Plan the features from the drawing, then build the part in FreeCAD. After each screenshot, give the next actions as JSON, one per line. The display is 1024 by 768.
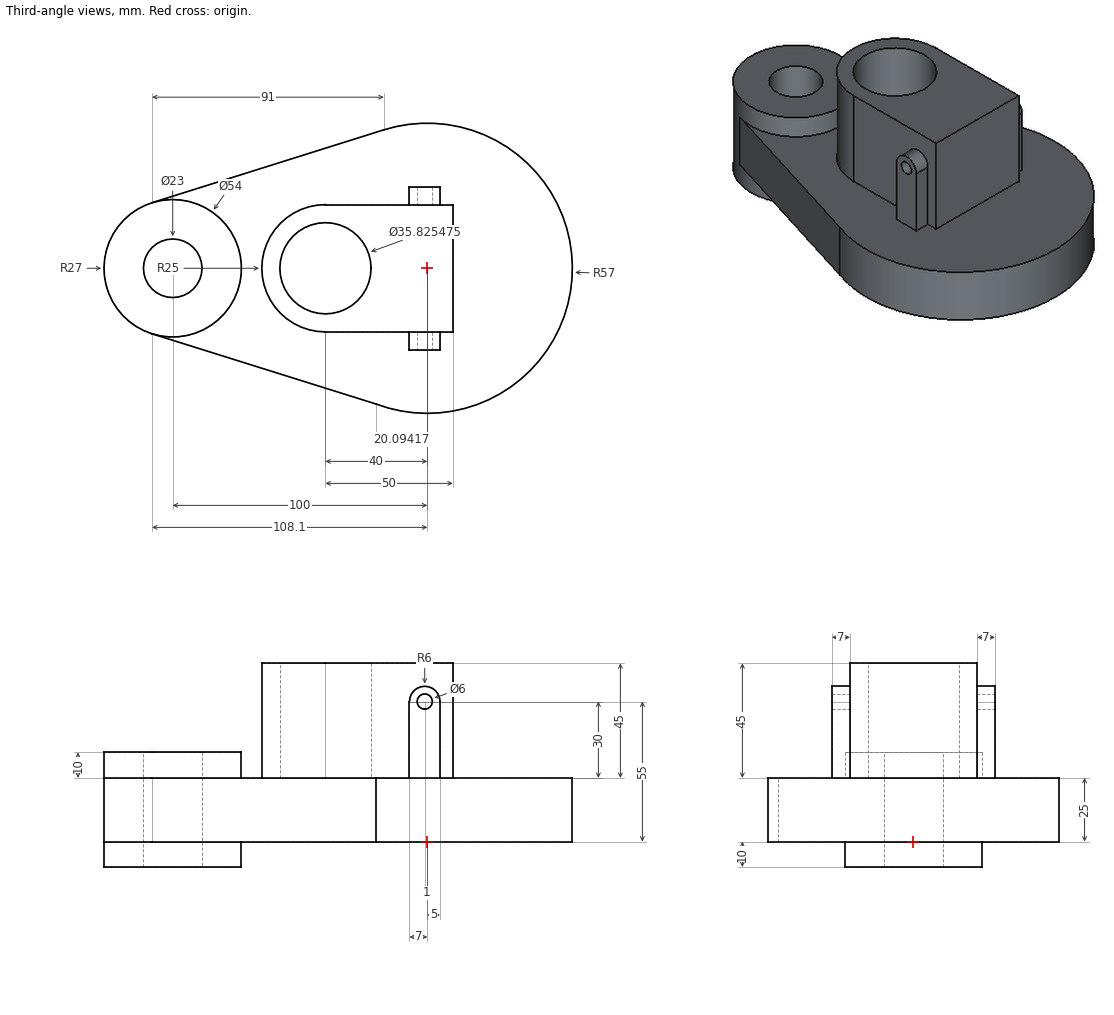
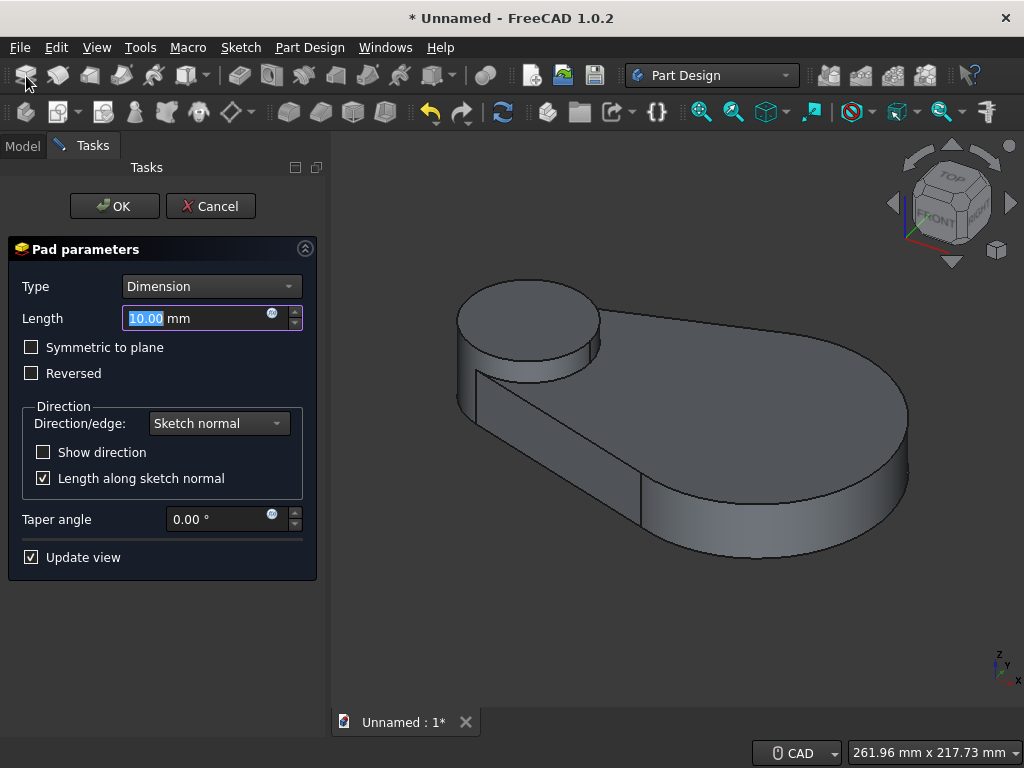
{"action": "type", "text": "10"}
{"action": "key", "text": "Tab"}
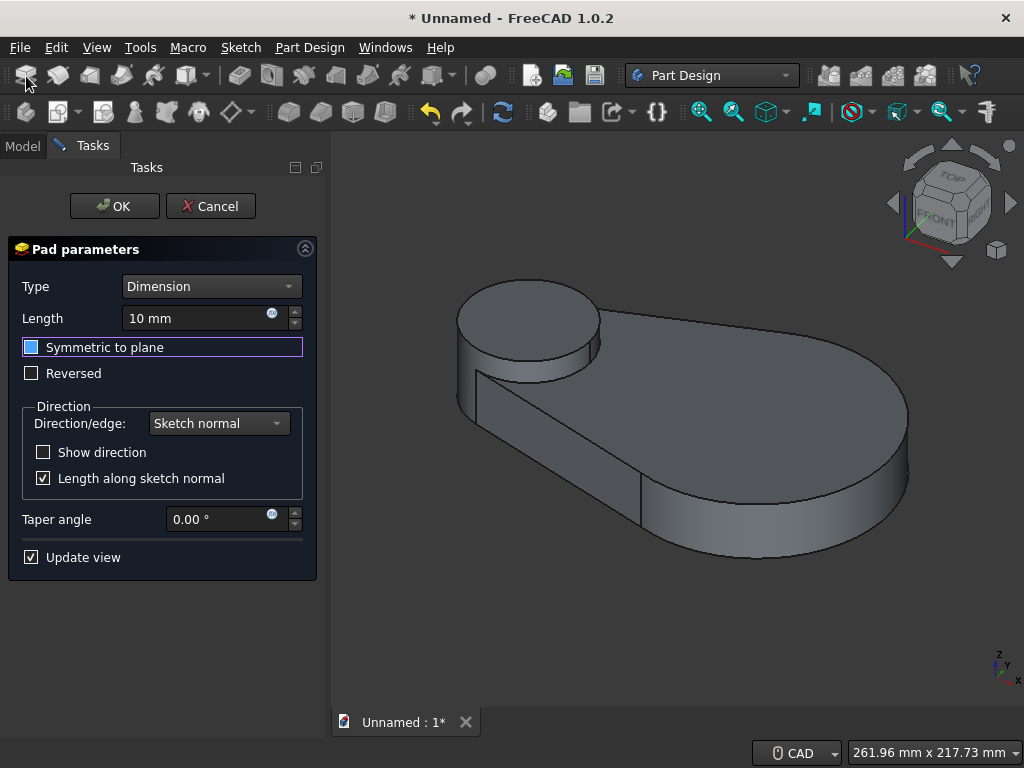
{"action": "left_click", "coordinate": [115, 206]}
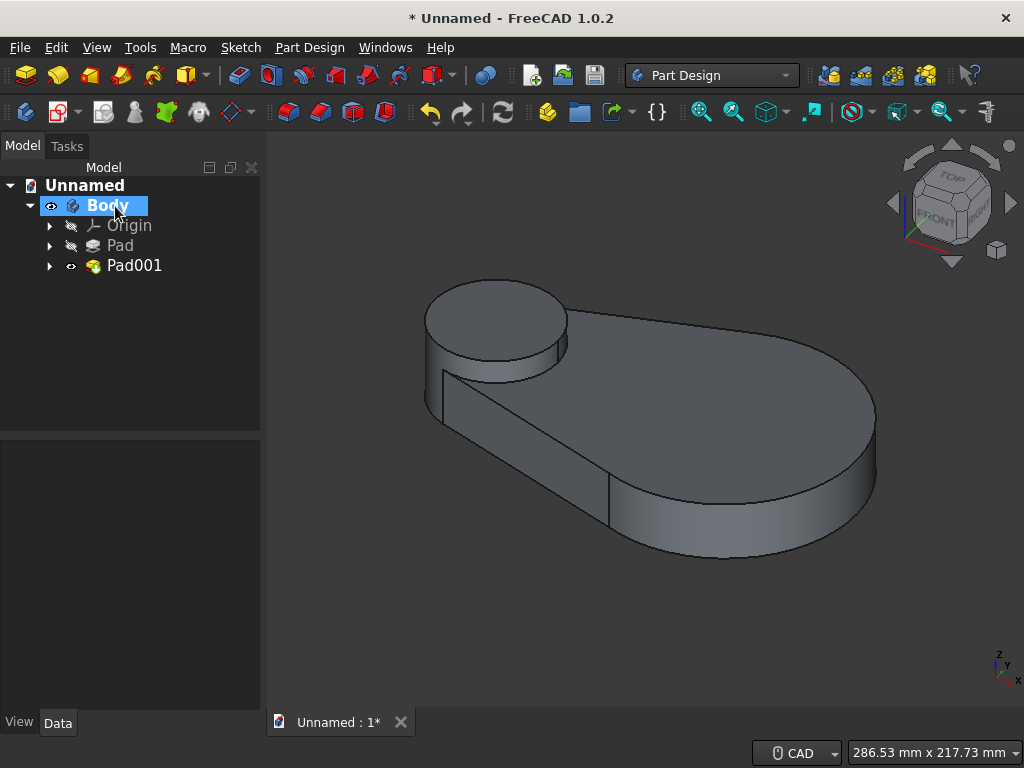
{"action": "left_click", "coordinate": [50, 226]}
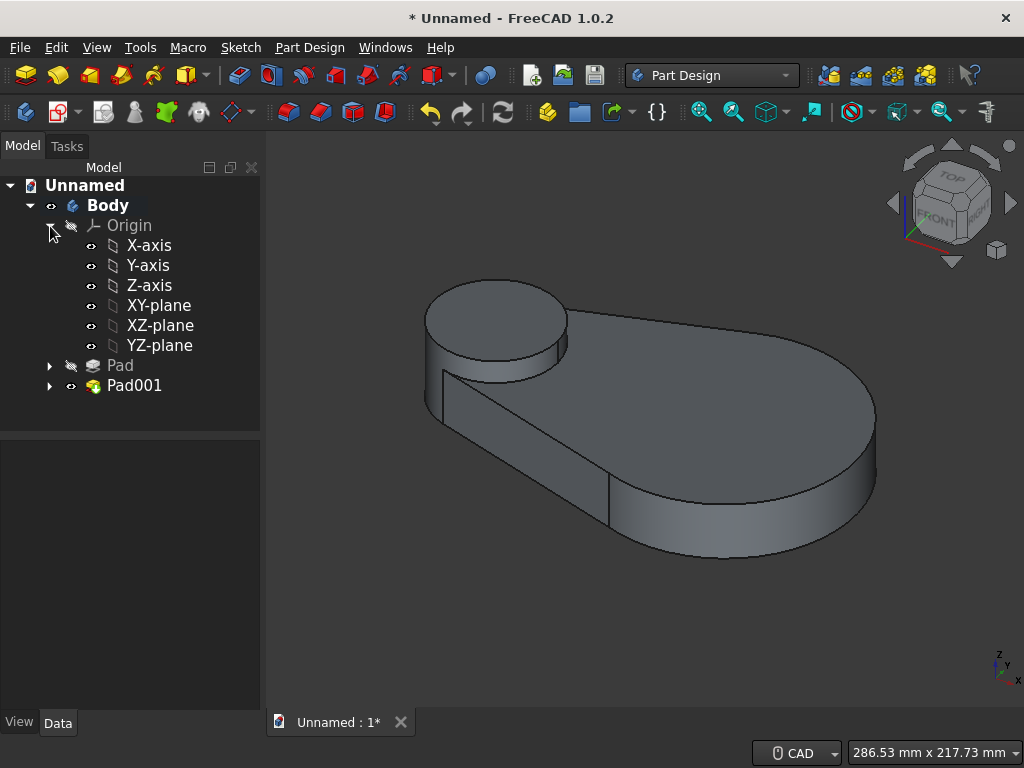
{"action": "left_click", "coordinate": [136, 306]}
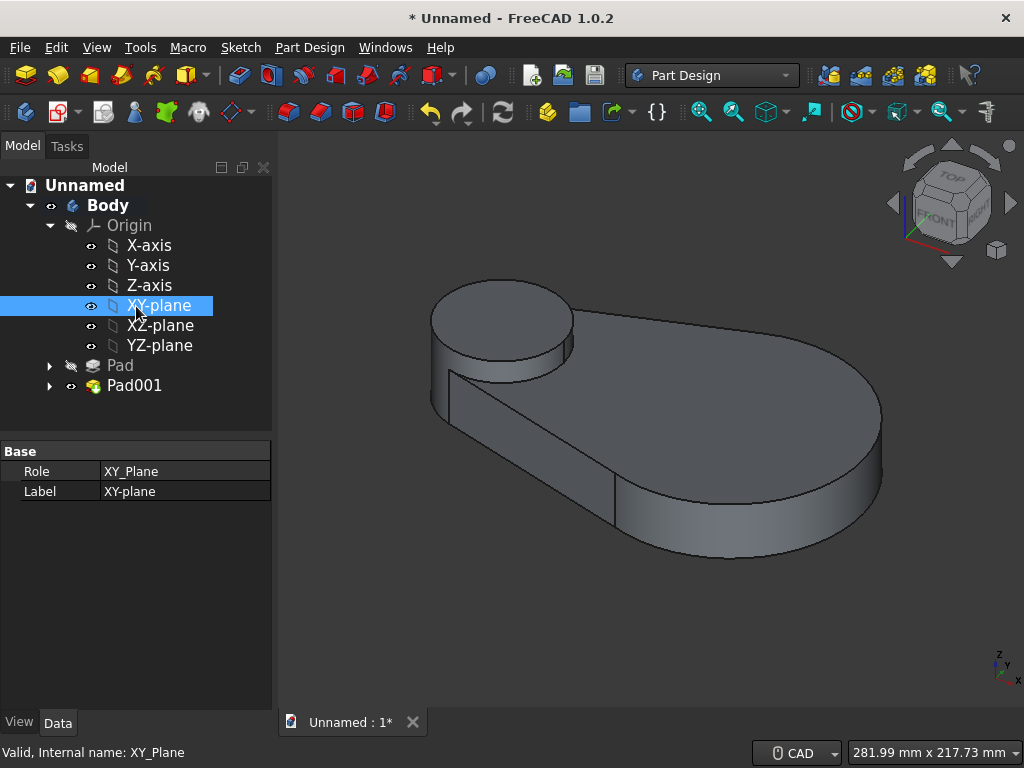
{"action": "left_click", "coordinate": [232, 112]}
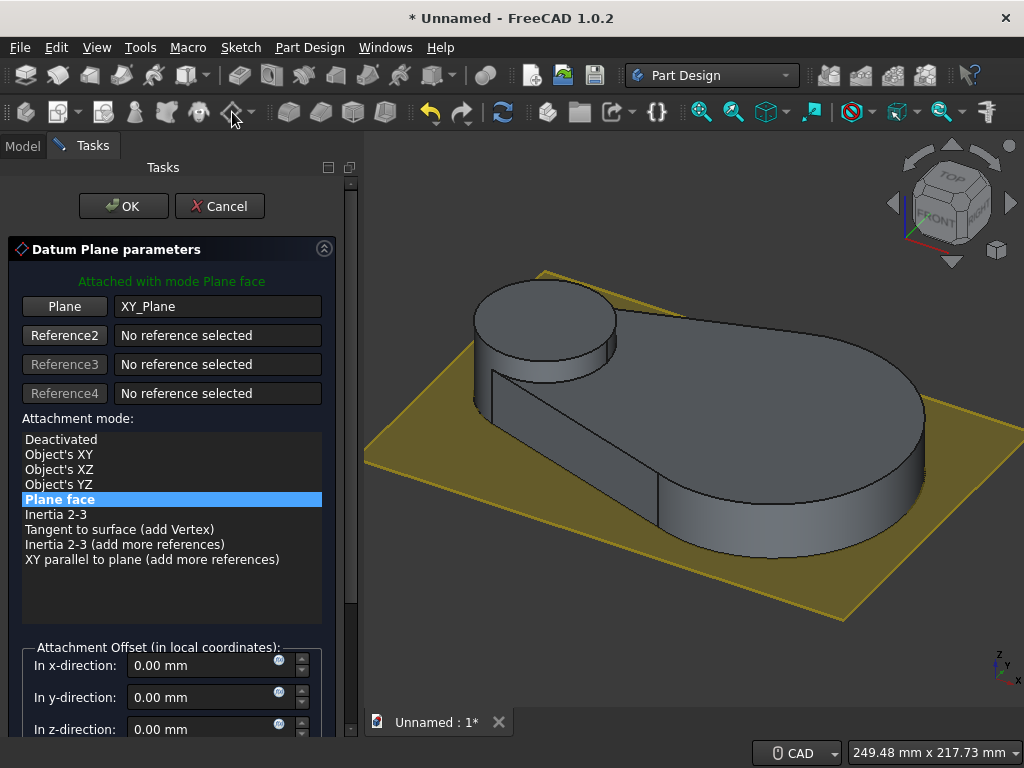
{"action": "scroll", "coordinate": [351, 456], "scroll_direction": "down", "scroll_amount": 2}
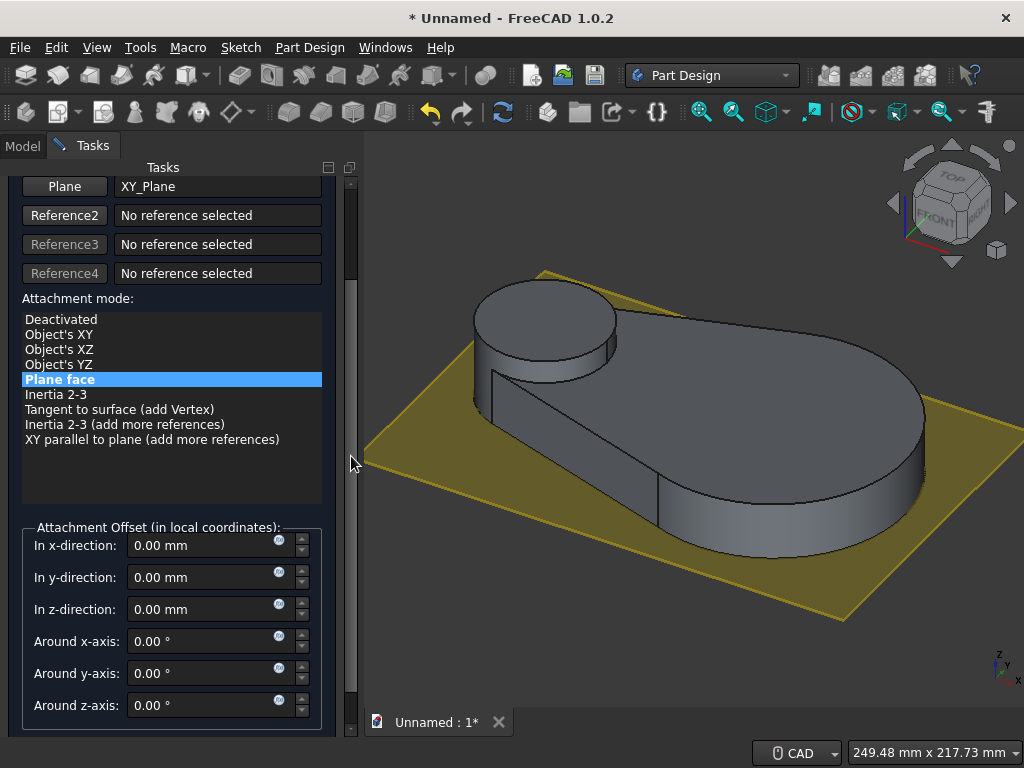
{"action": "triple_click", "coordinate": [210, 609]}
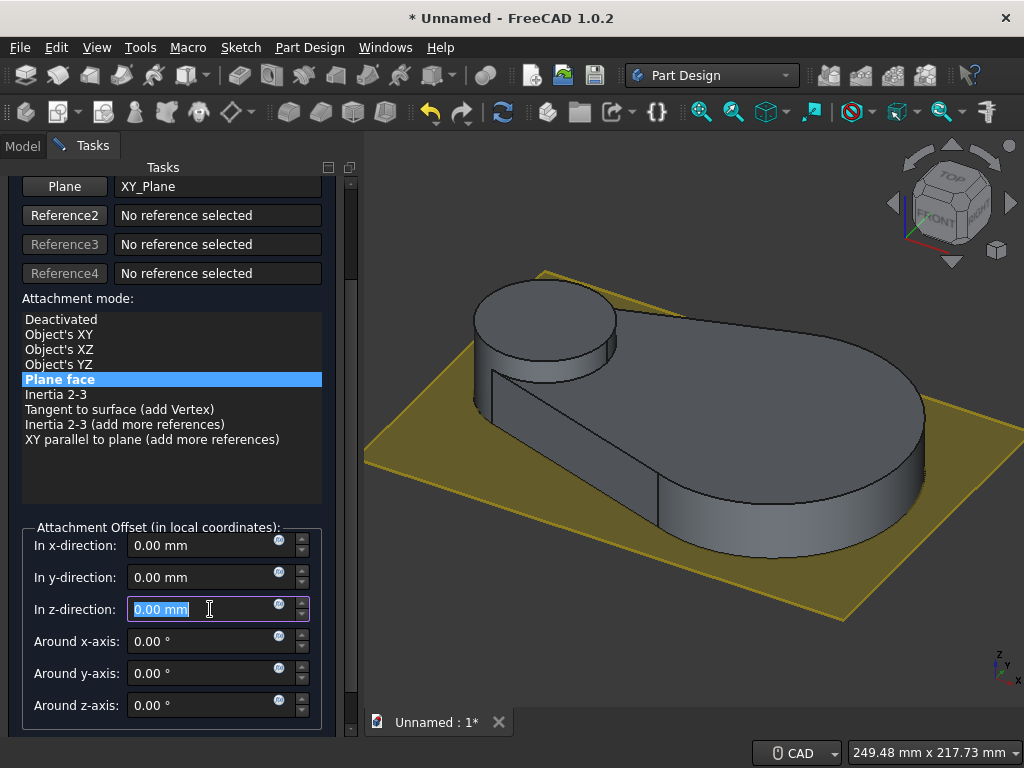
{"action": "type", "text": "-10"}
{"action": "key", "text": "Tab"}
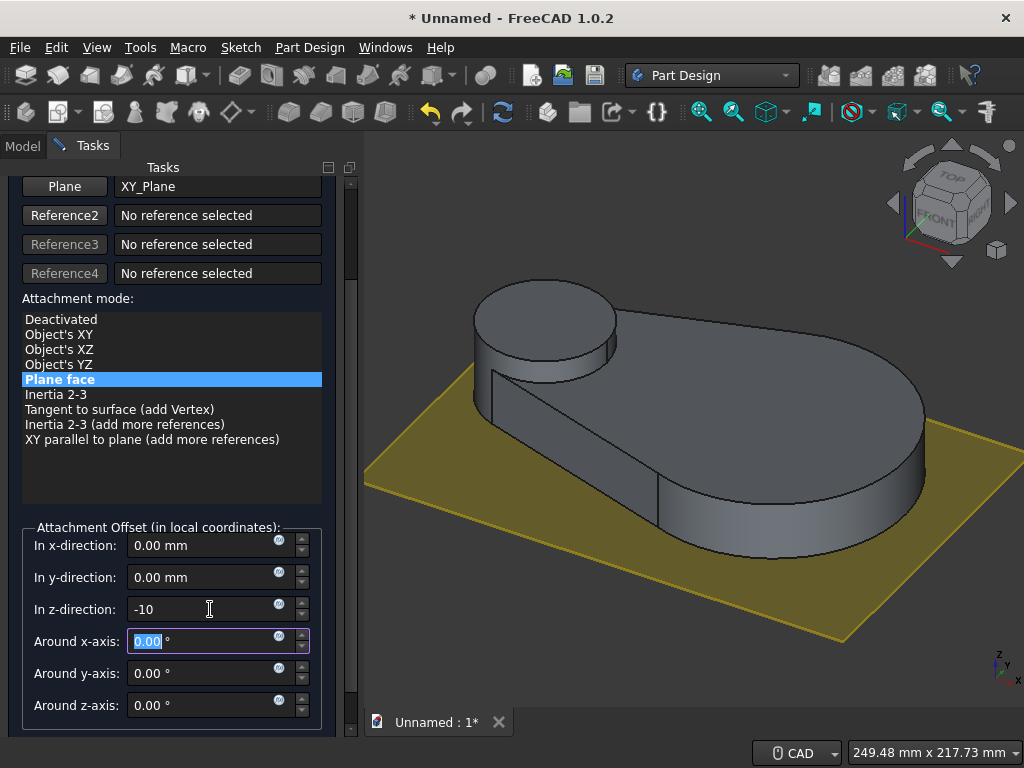
{"action": "scroll", "coordinate": [351, 456], "scroll_direction": "up", "scroll_amount": 3}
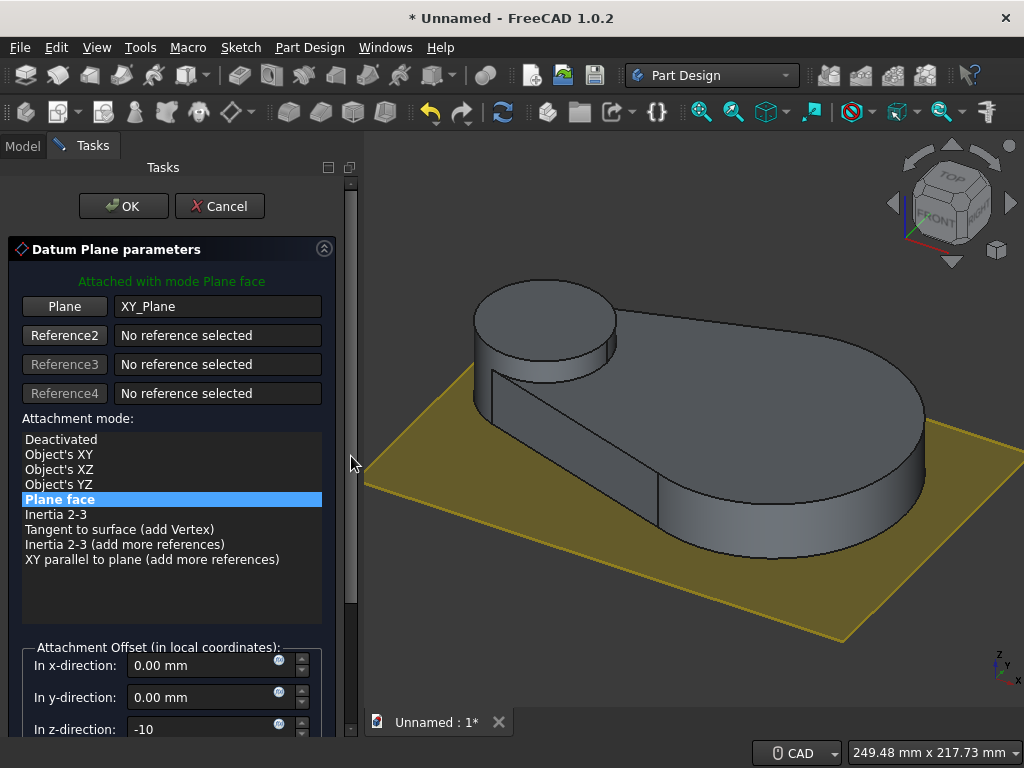
{"action": "left_click", "coordinate": [124, 206]}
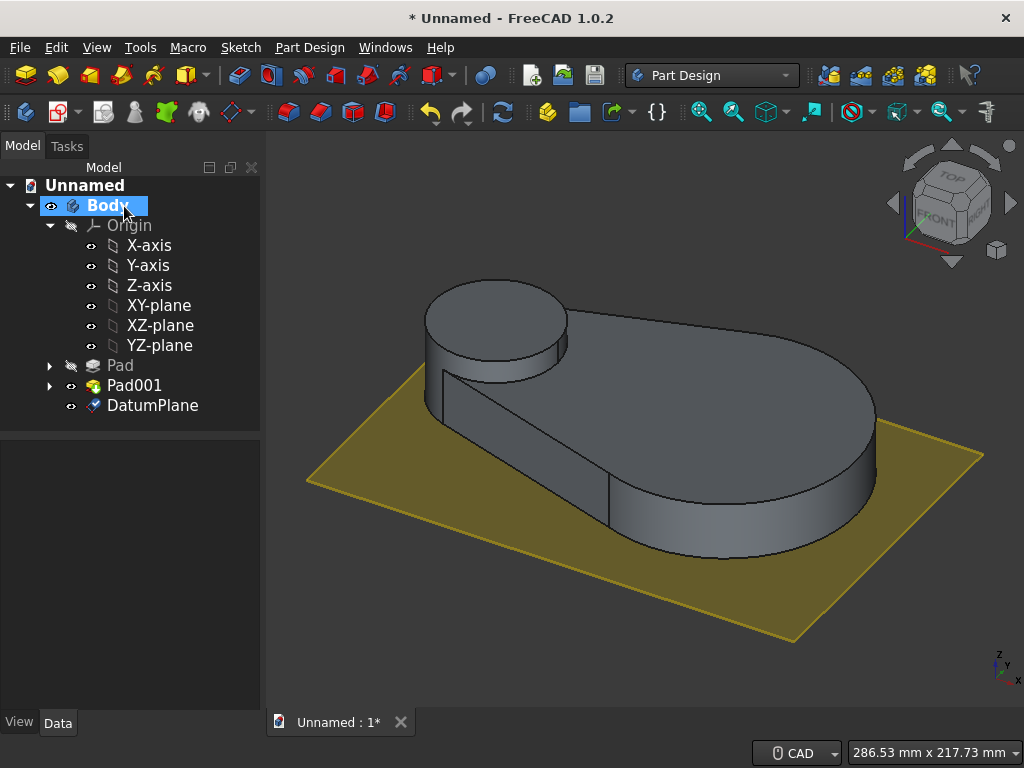
{"action": "left_click", "coordinate": [116, 406]}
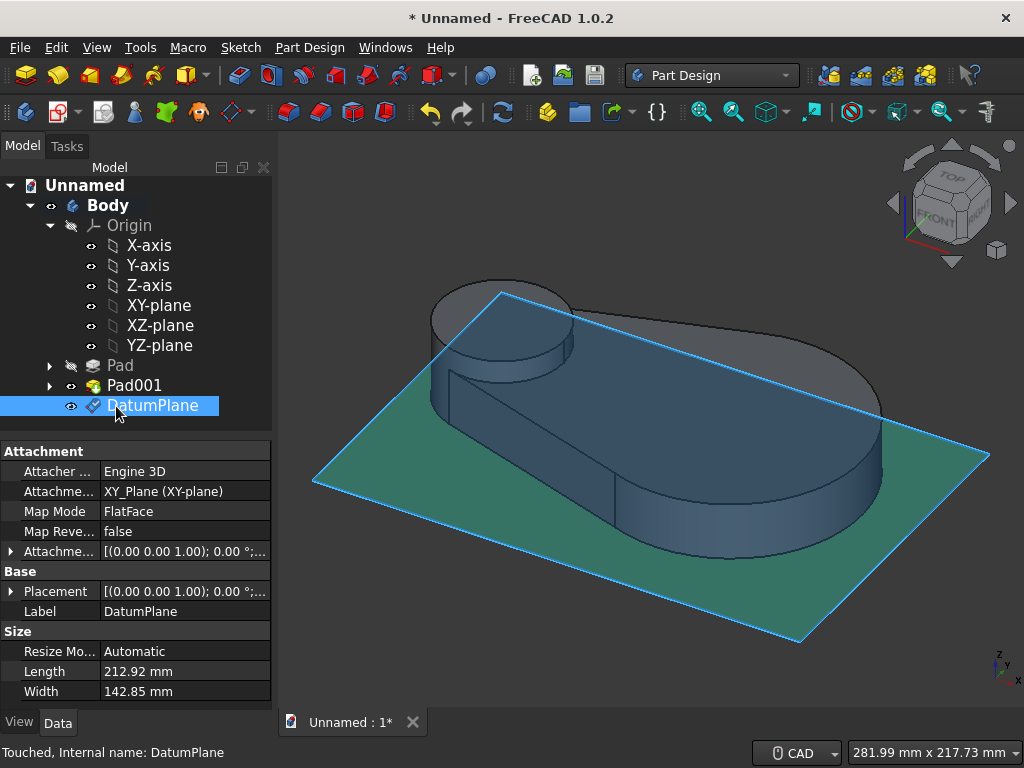
{"action": "left_click", "coordinate": [58, 112]}